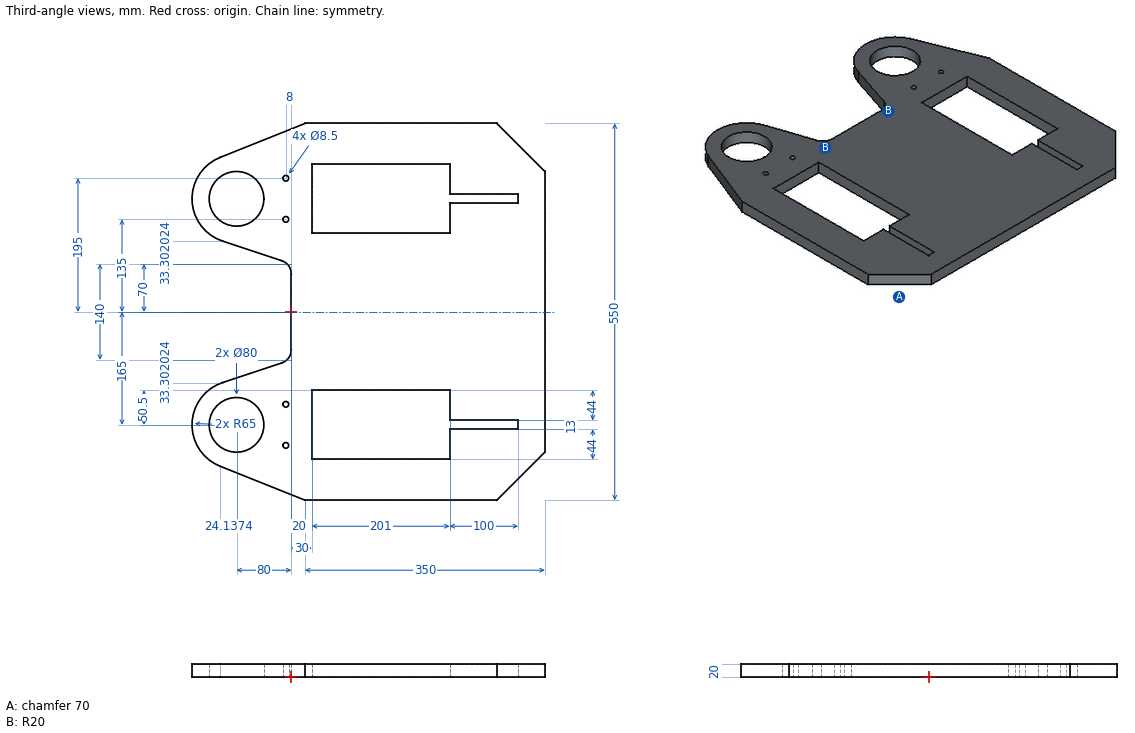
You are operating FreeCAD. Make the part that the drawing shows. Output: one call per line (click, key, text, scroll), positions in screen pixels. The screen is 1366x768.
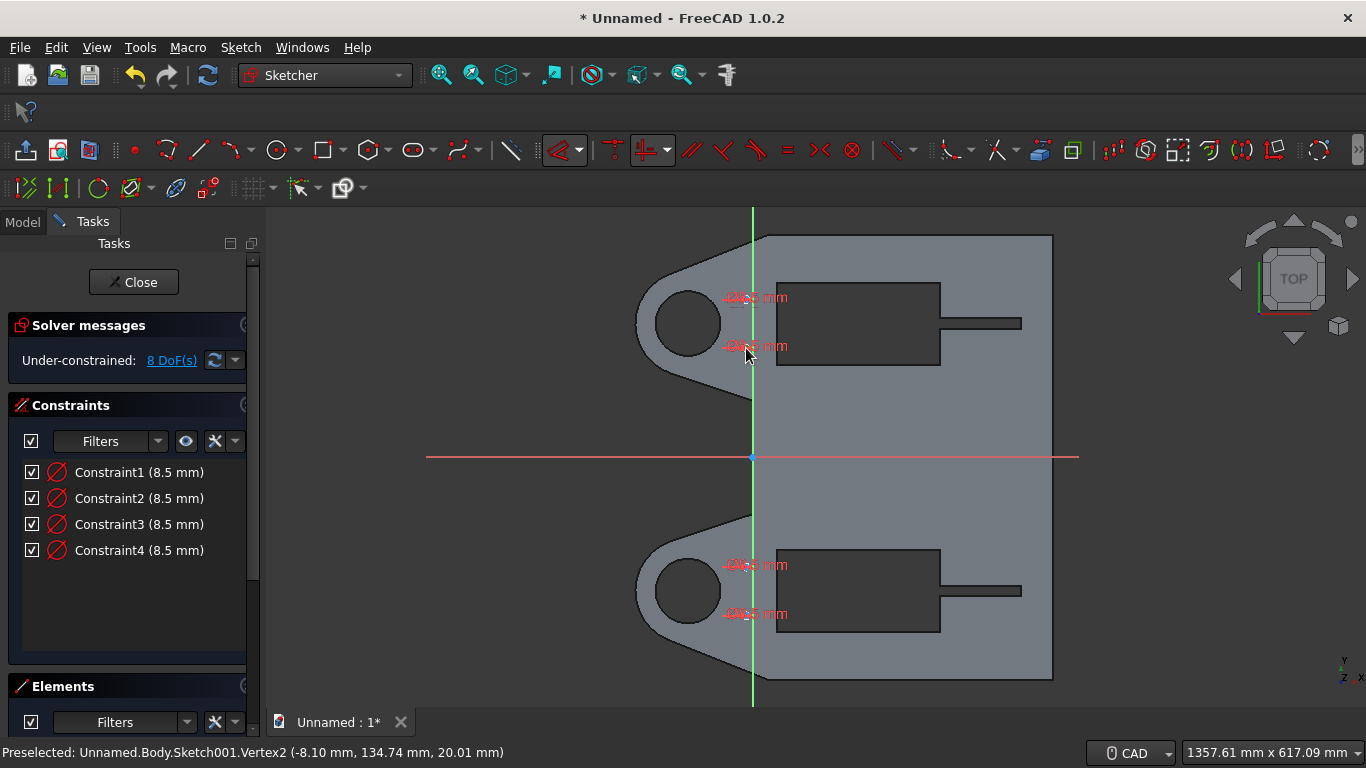
click(746, 567)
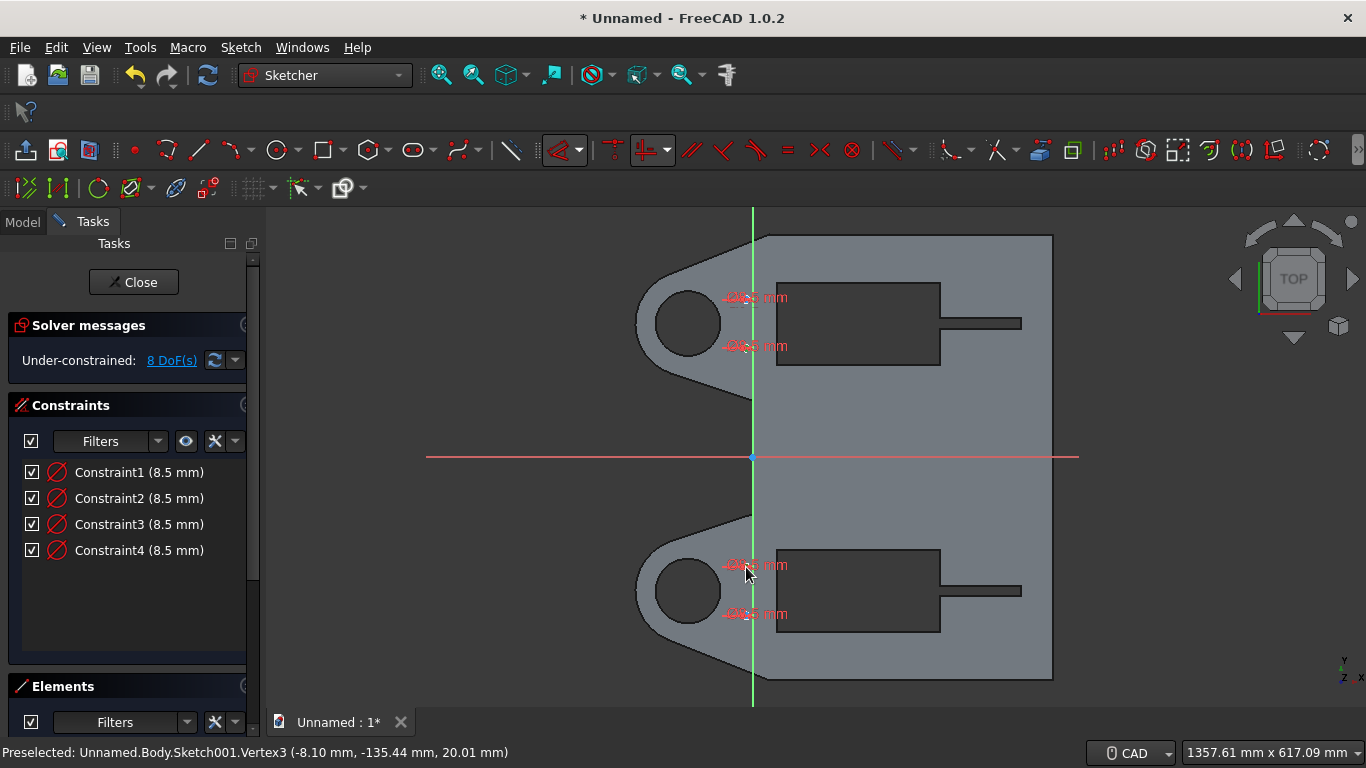
click(424, 457)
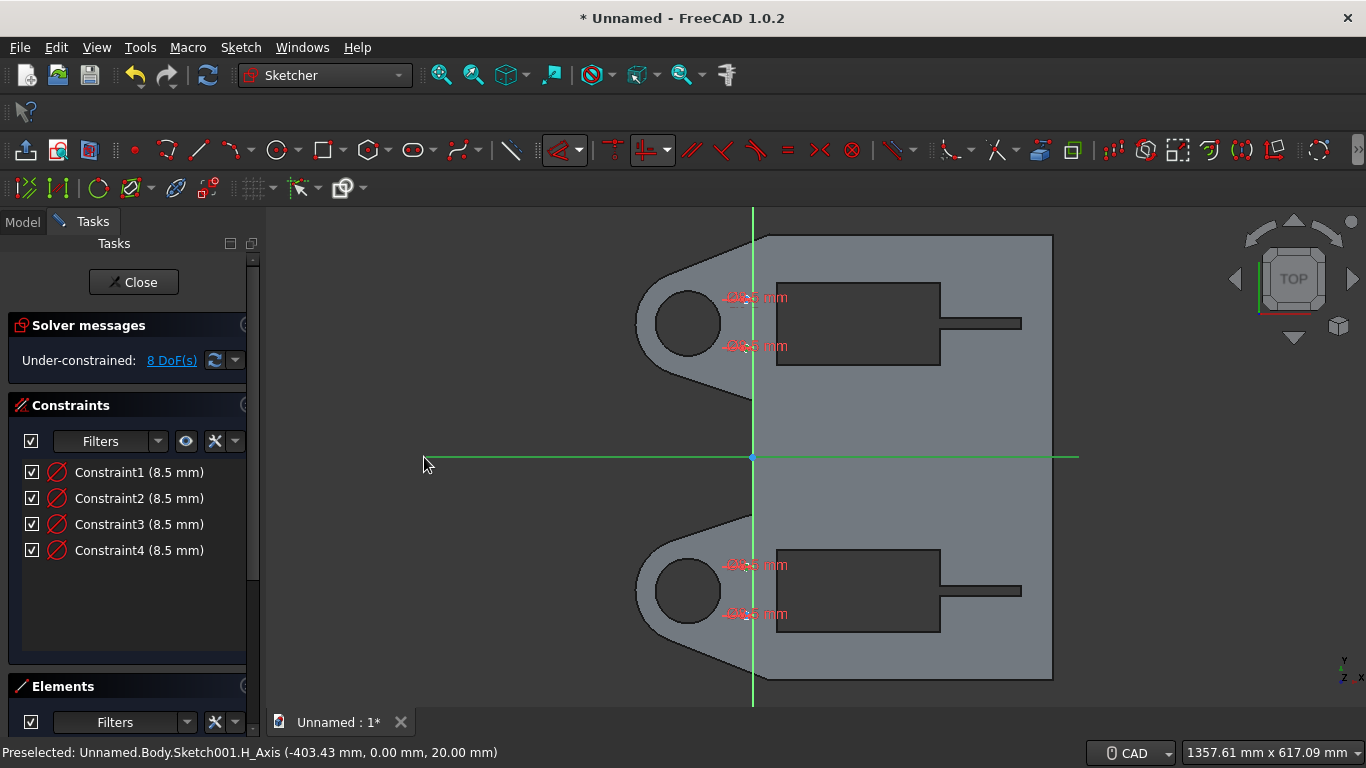
key(s)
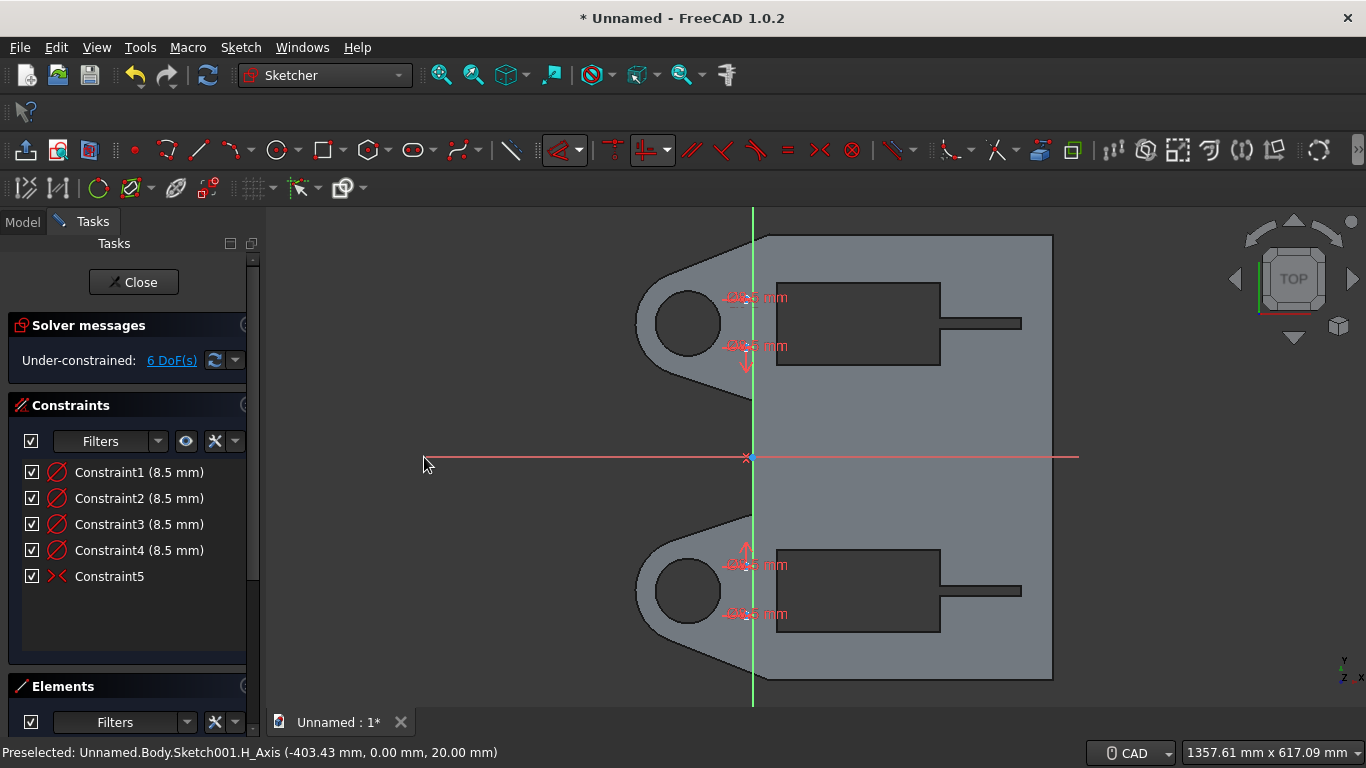
click(746, 300)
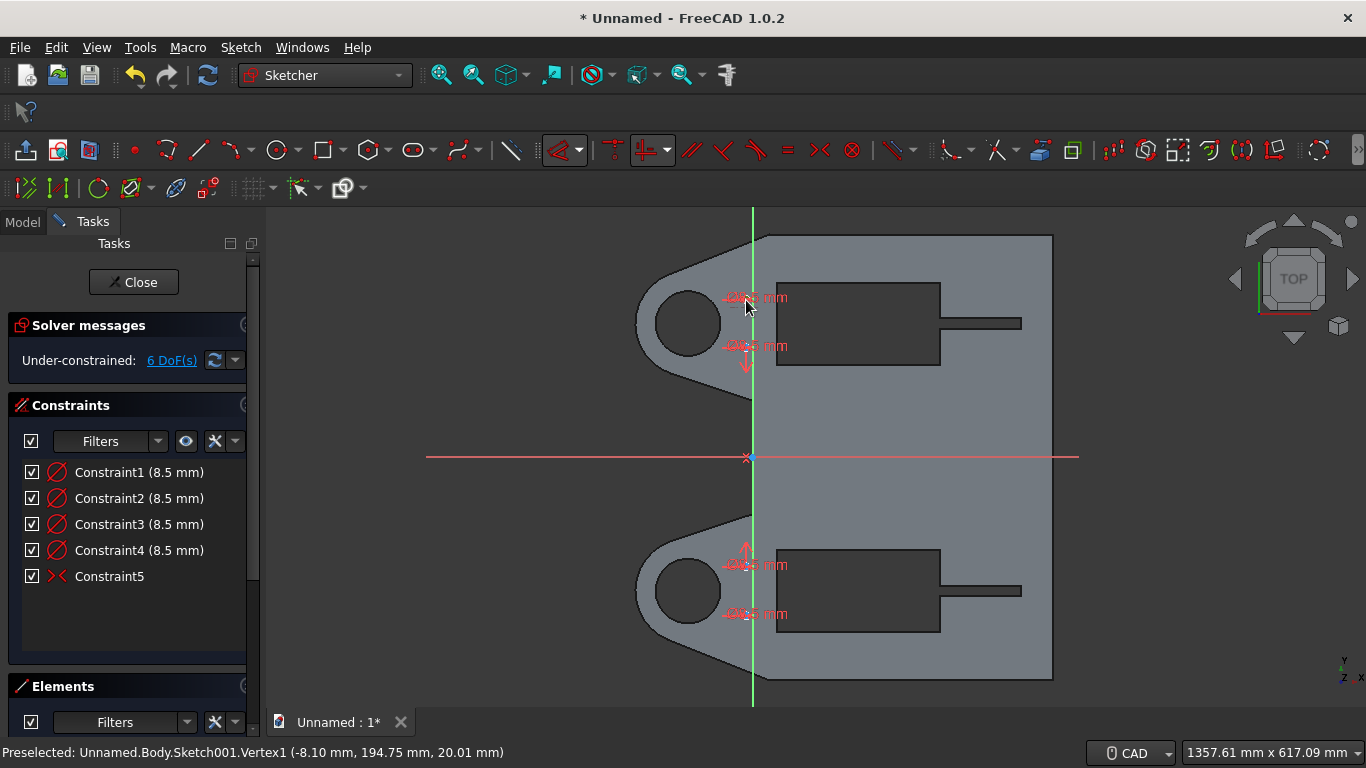
click(746, 616)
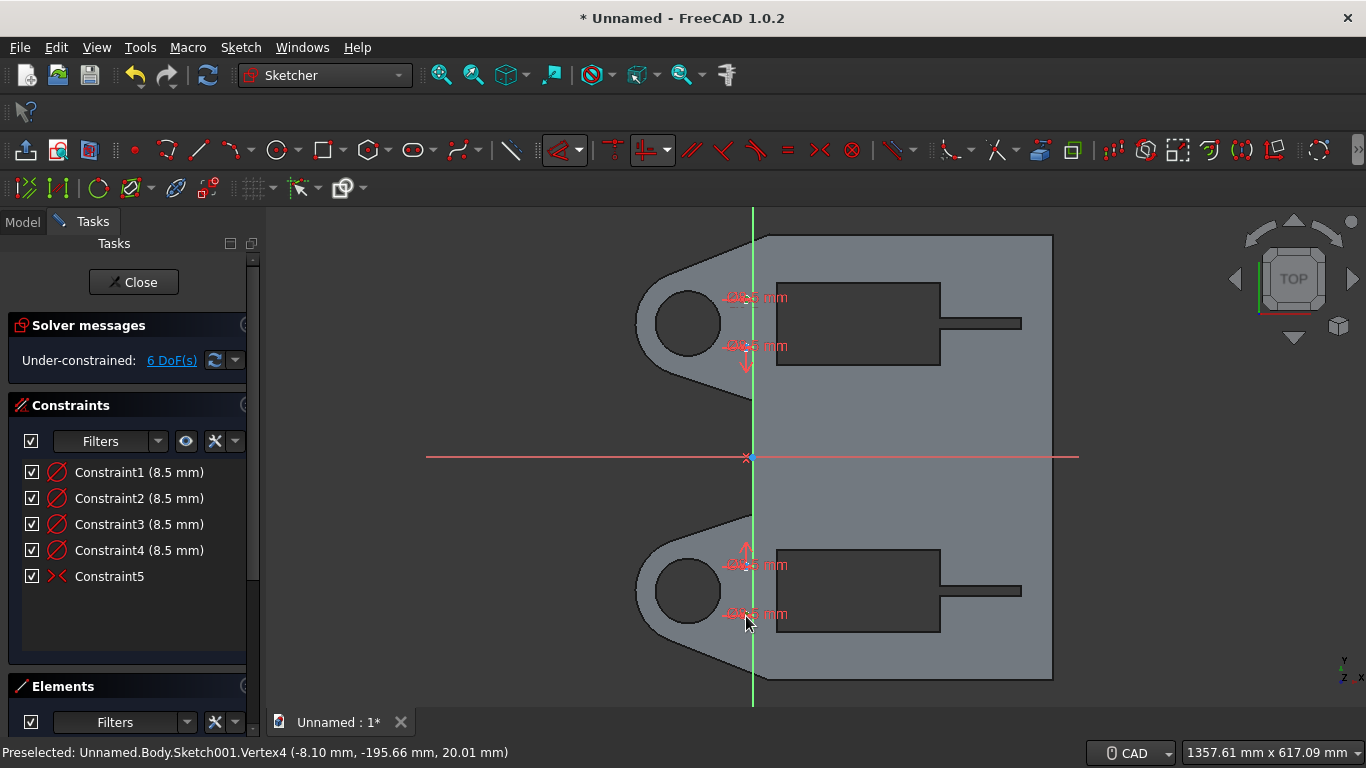
click(424, 457)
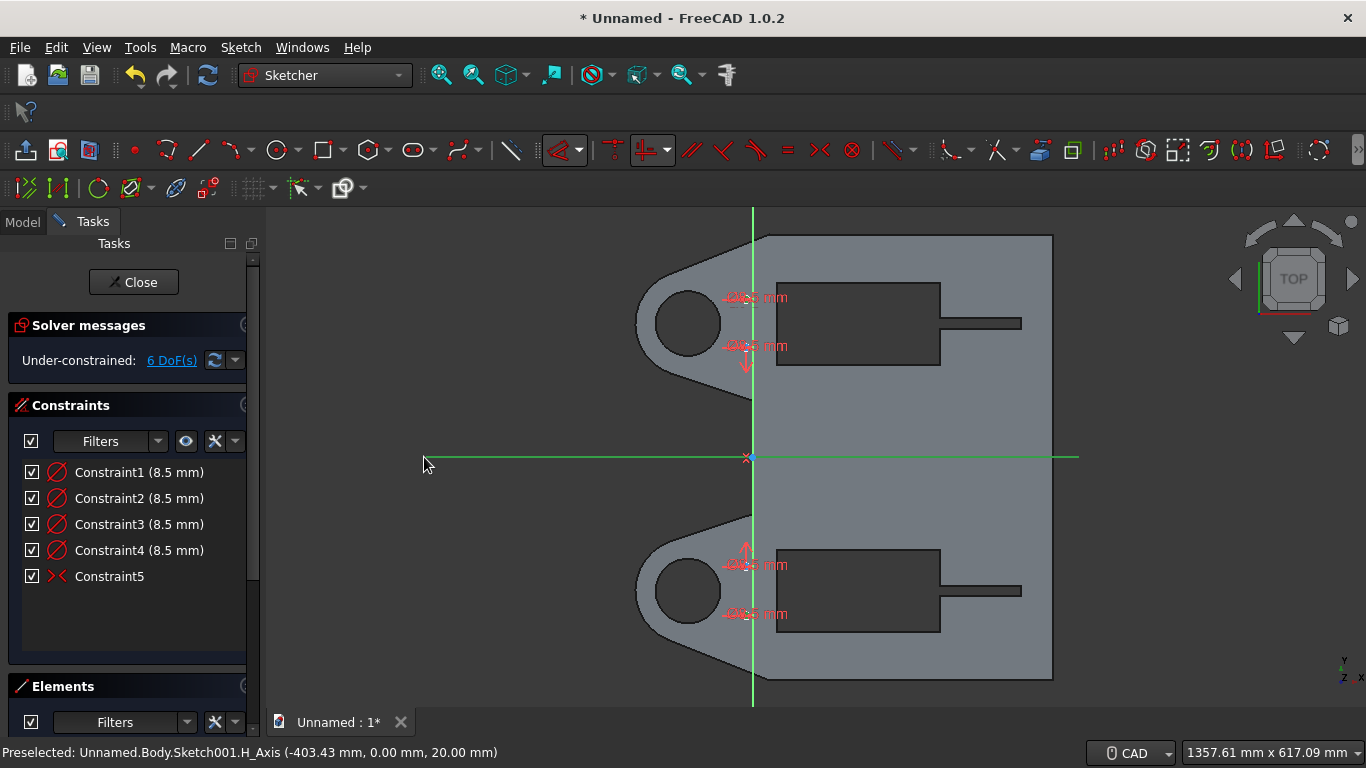
key(s)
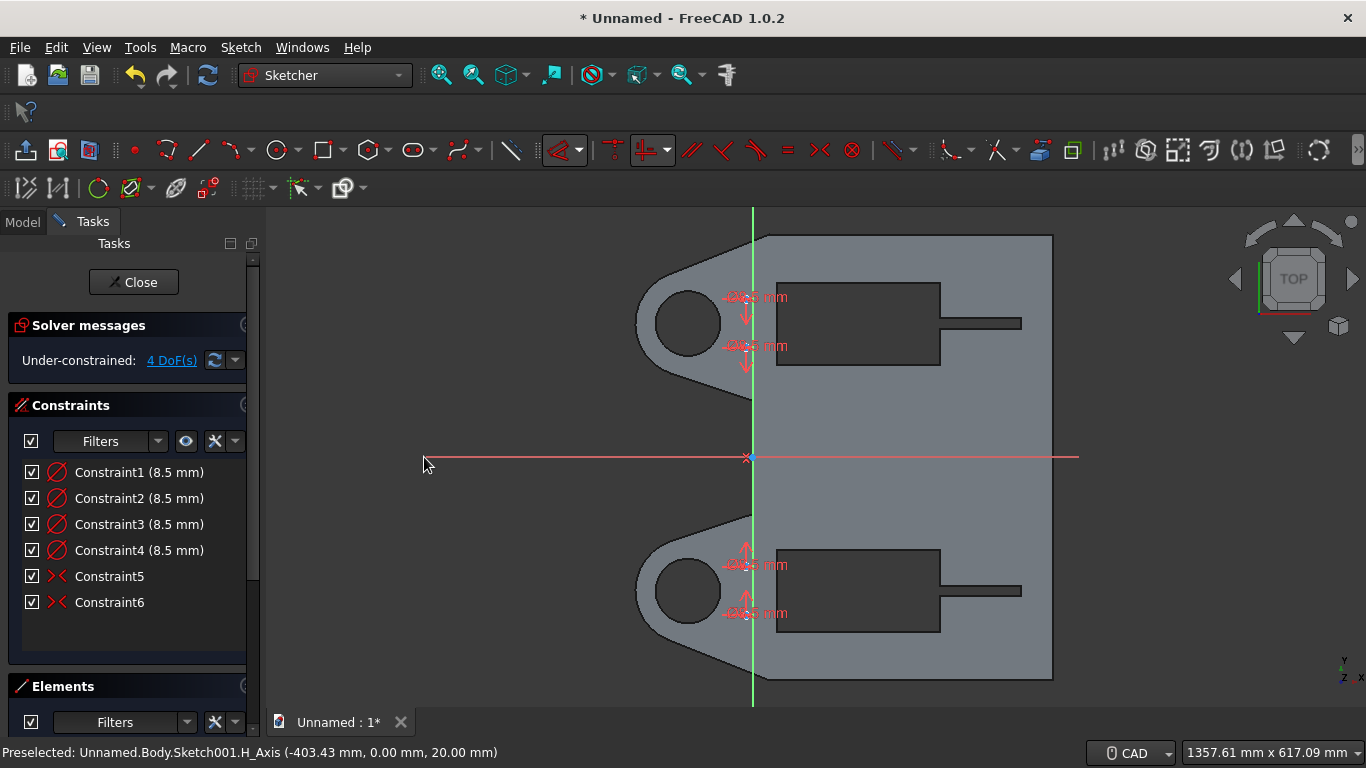
scroll(746, 299, up, 10)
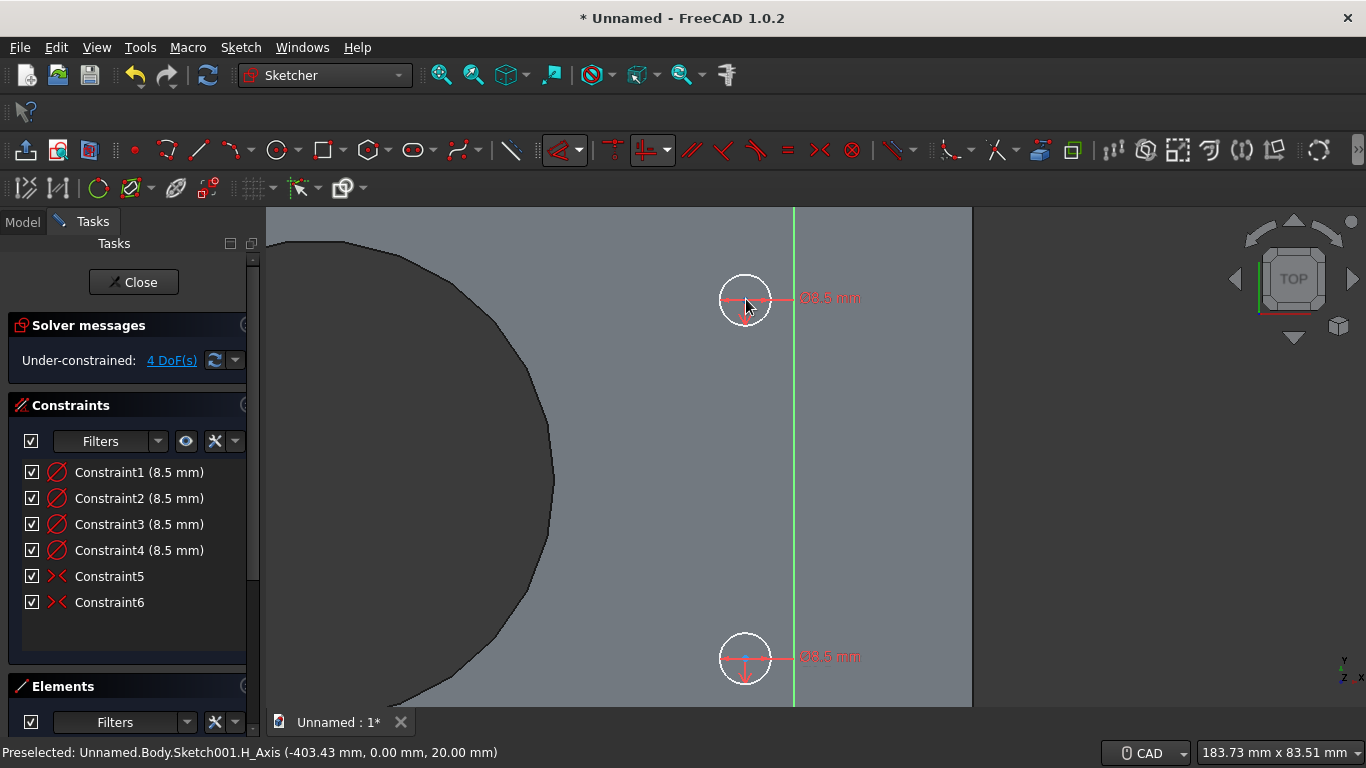
click(745, 300)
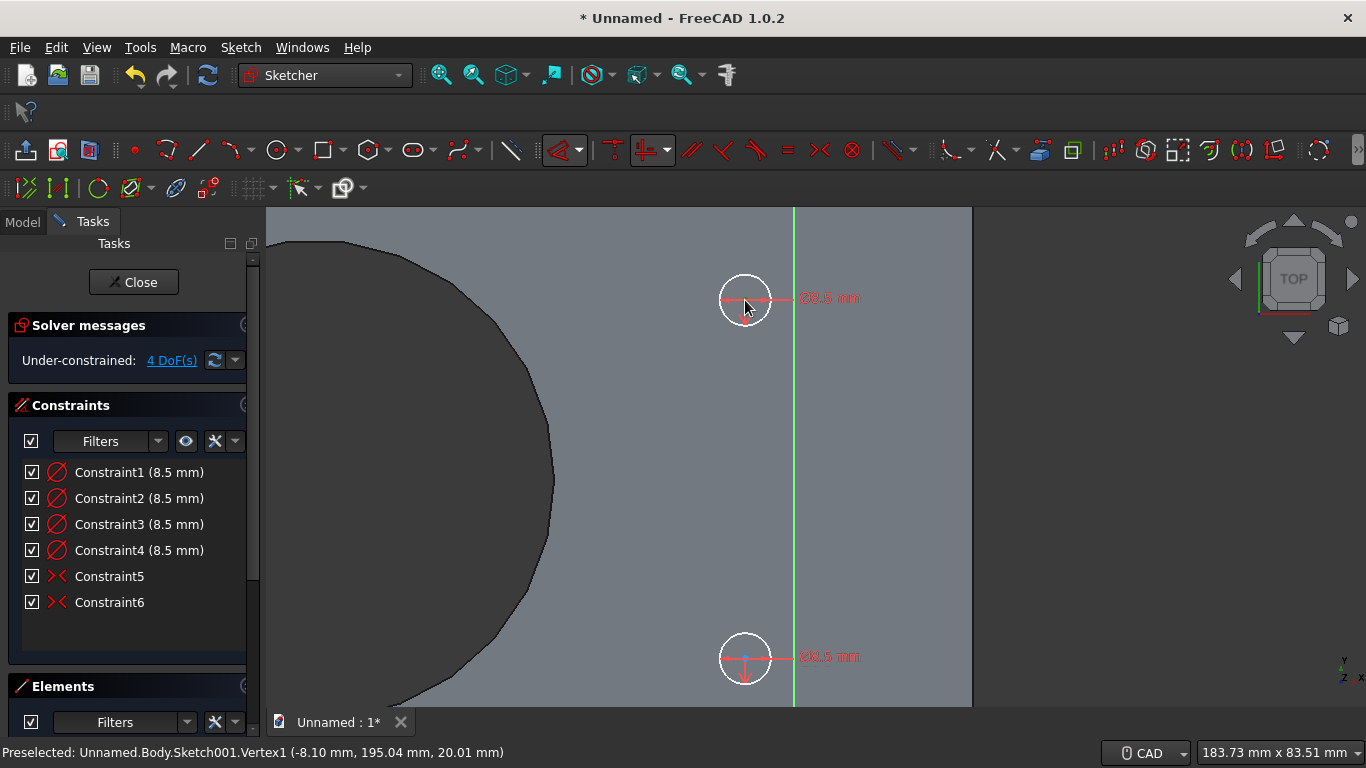
key(l)